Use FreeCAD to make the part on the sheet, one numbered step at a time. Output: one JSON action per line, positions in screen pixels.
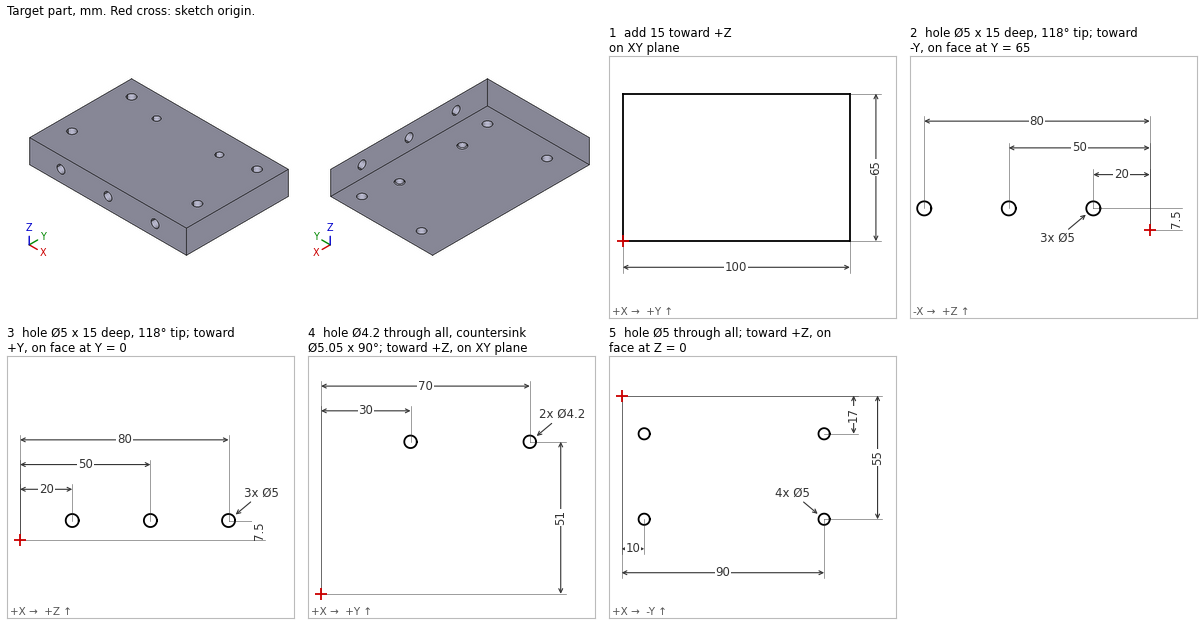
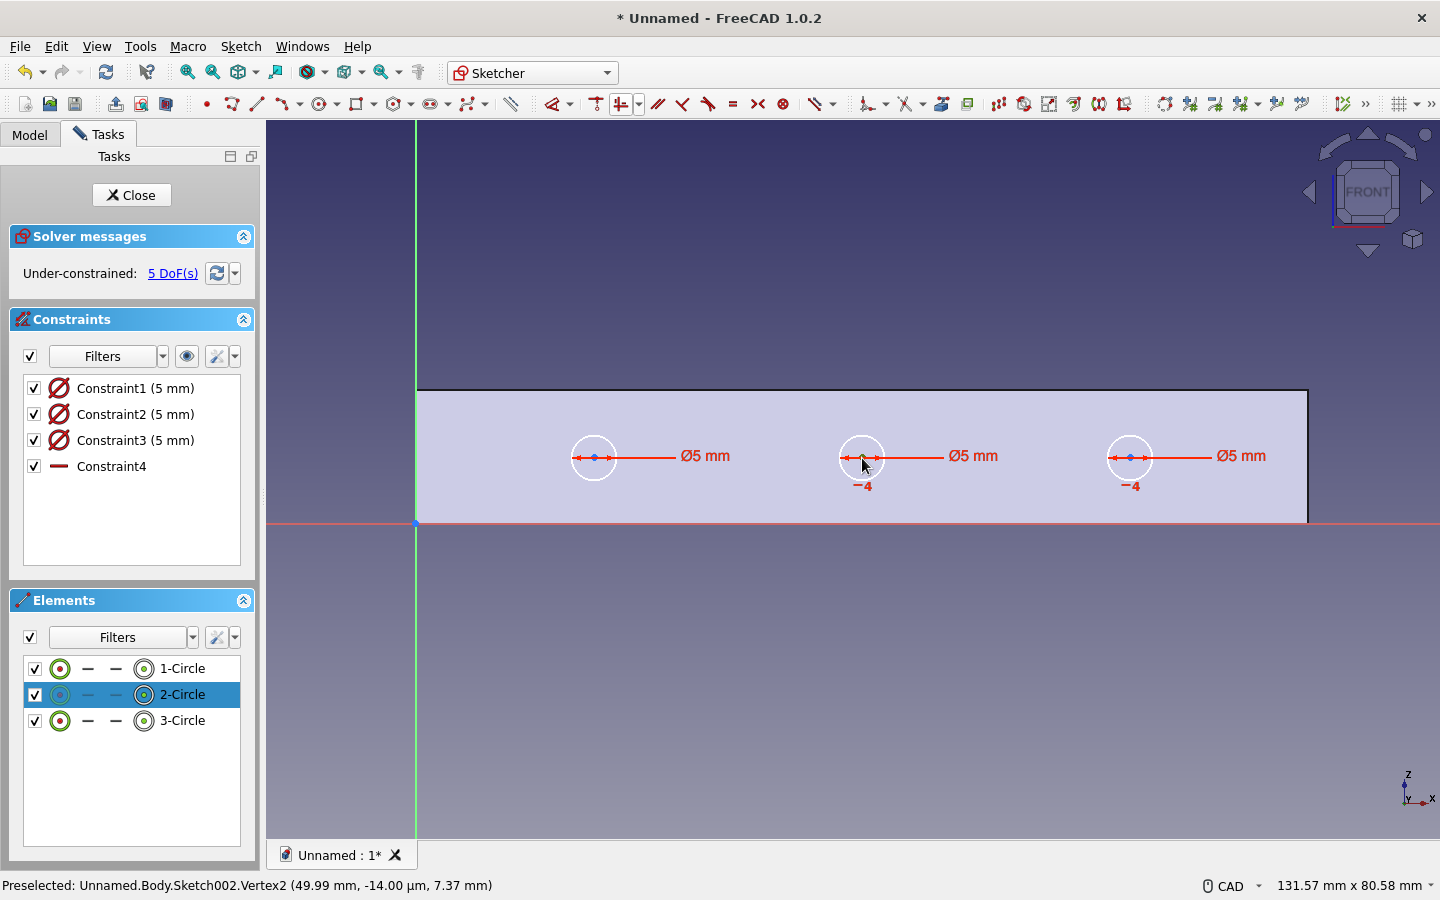
{"action": "left_click", "coordinate": [594, 458]}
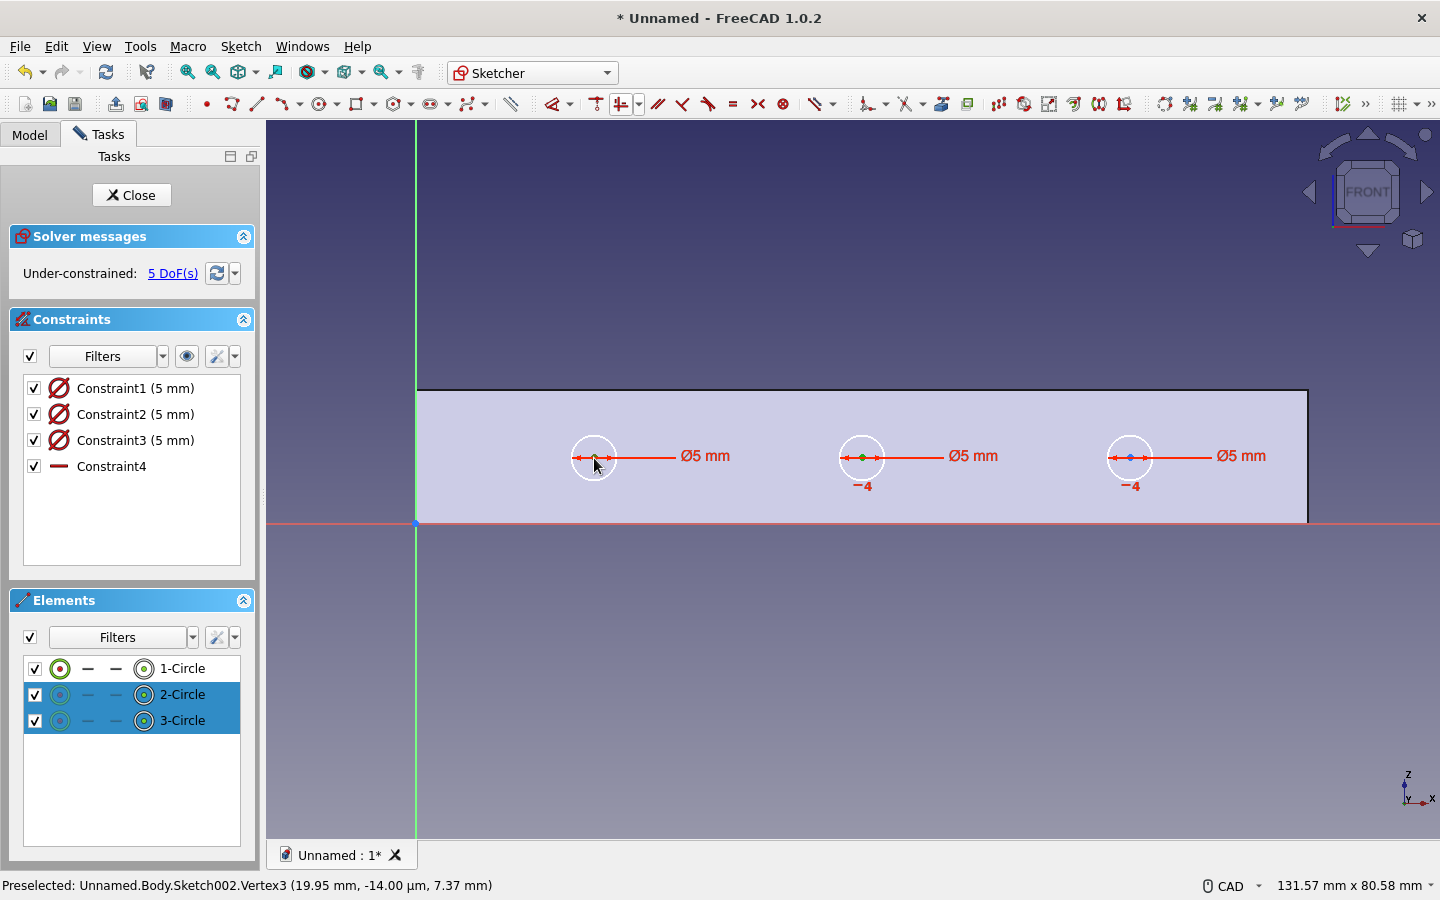
{"action": "key", "text": "h"}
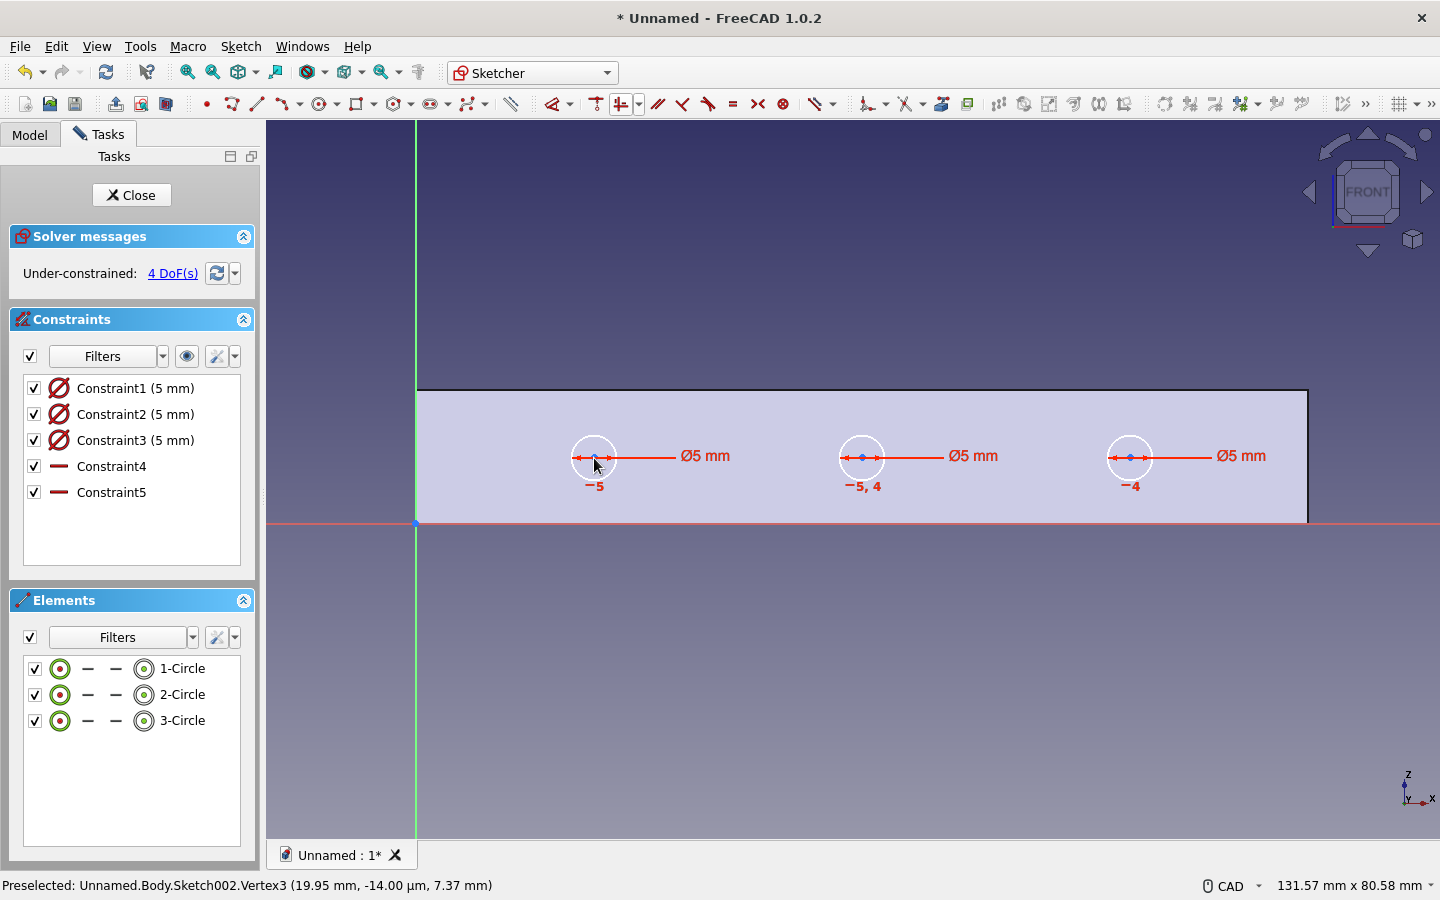
{"action": "left_click", "coordinate": [552, 104]}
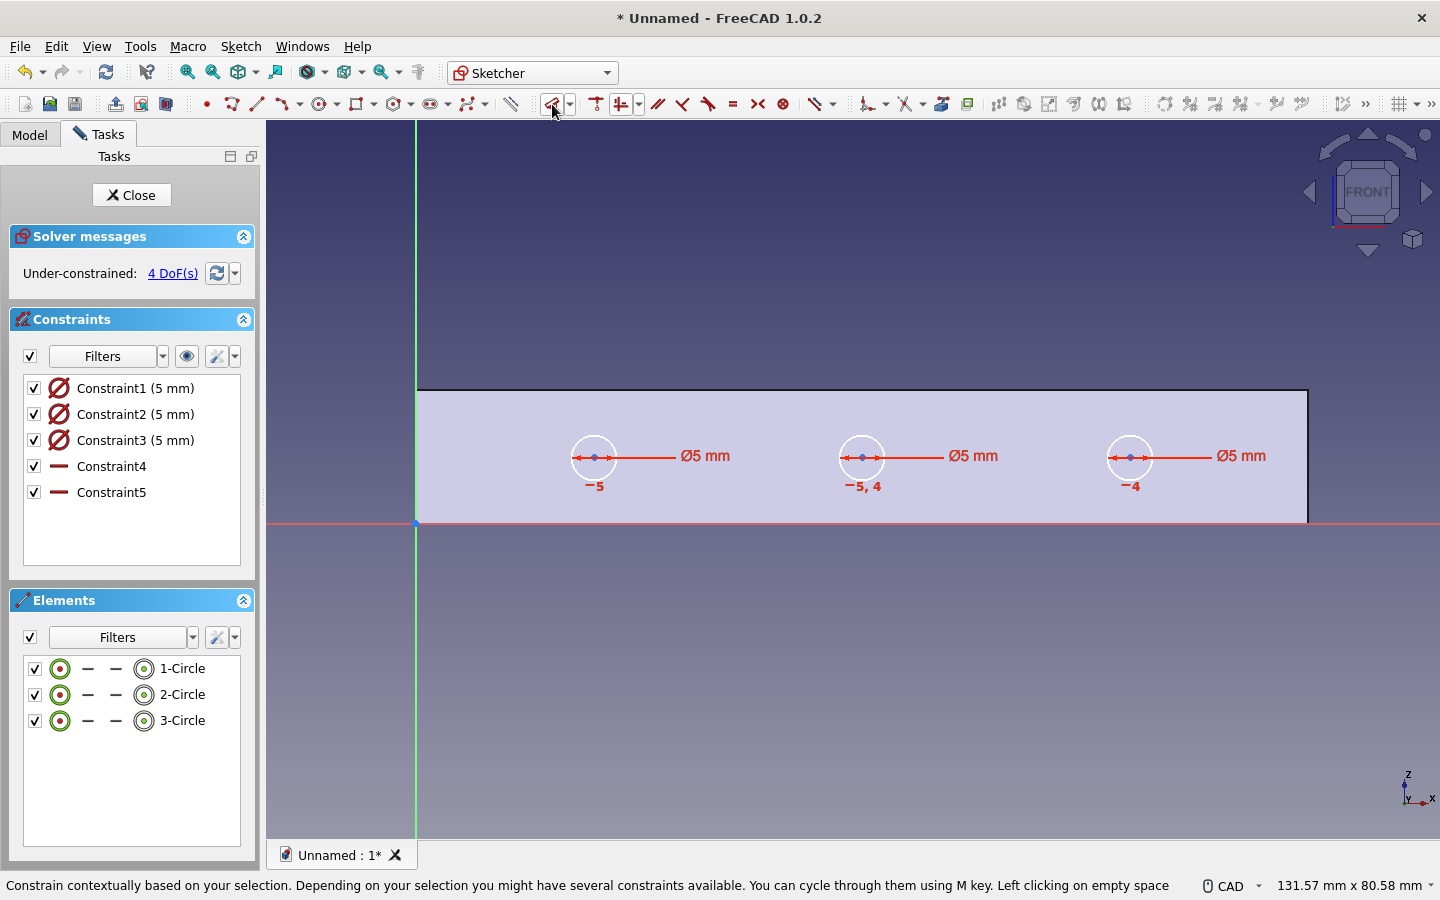
{"action": "left_click", "coordinate": [1130, 458]}
{"action": "left_click", "coordinate": [773, 558]}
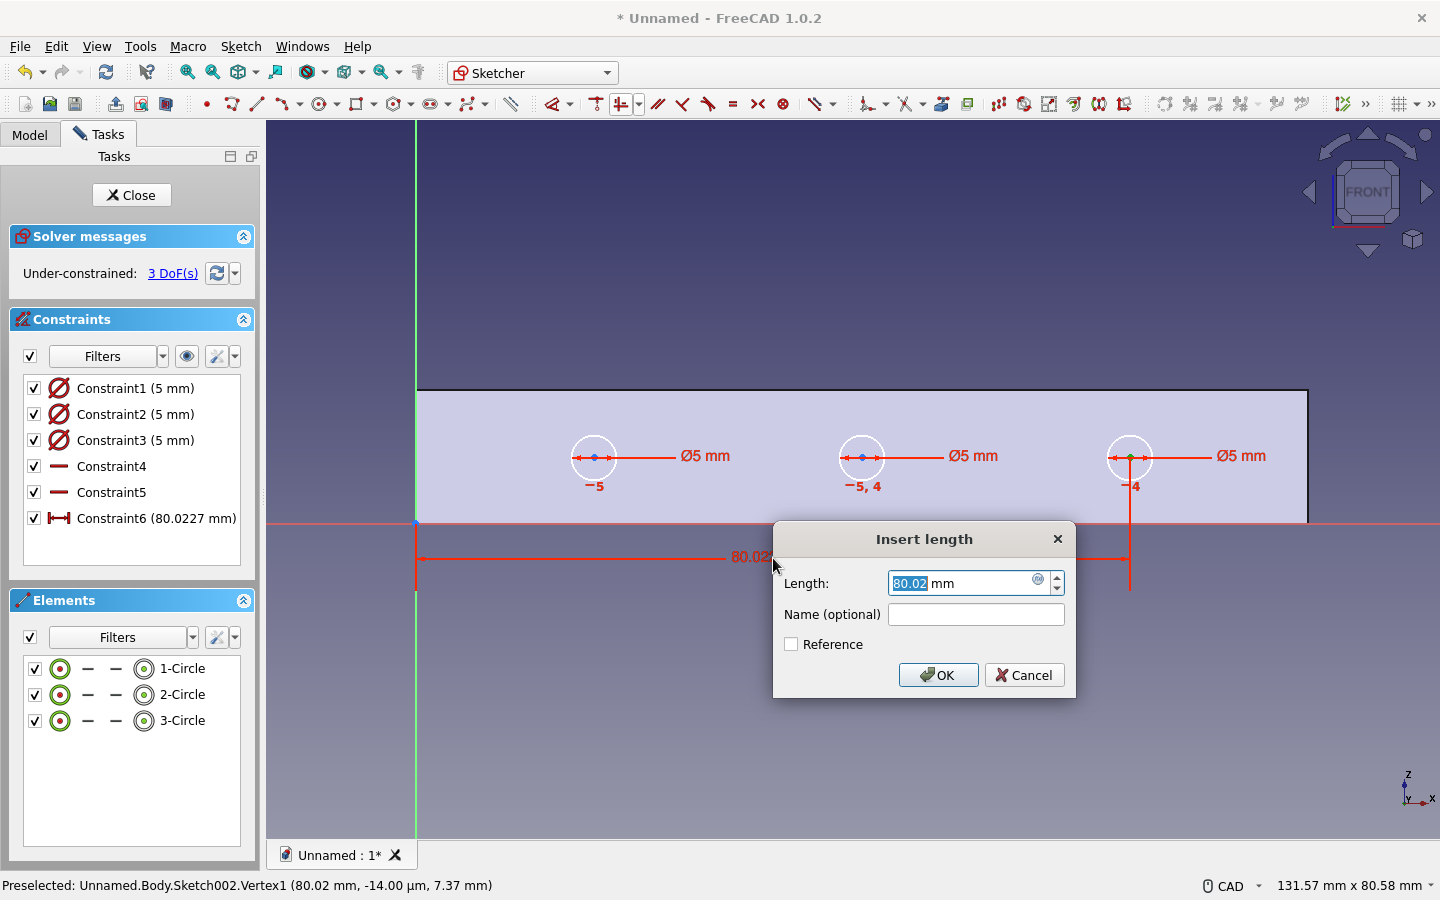
{"action": "type", "text": "80"}
{"action": "key", "text": "Return"}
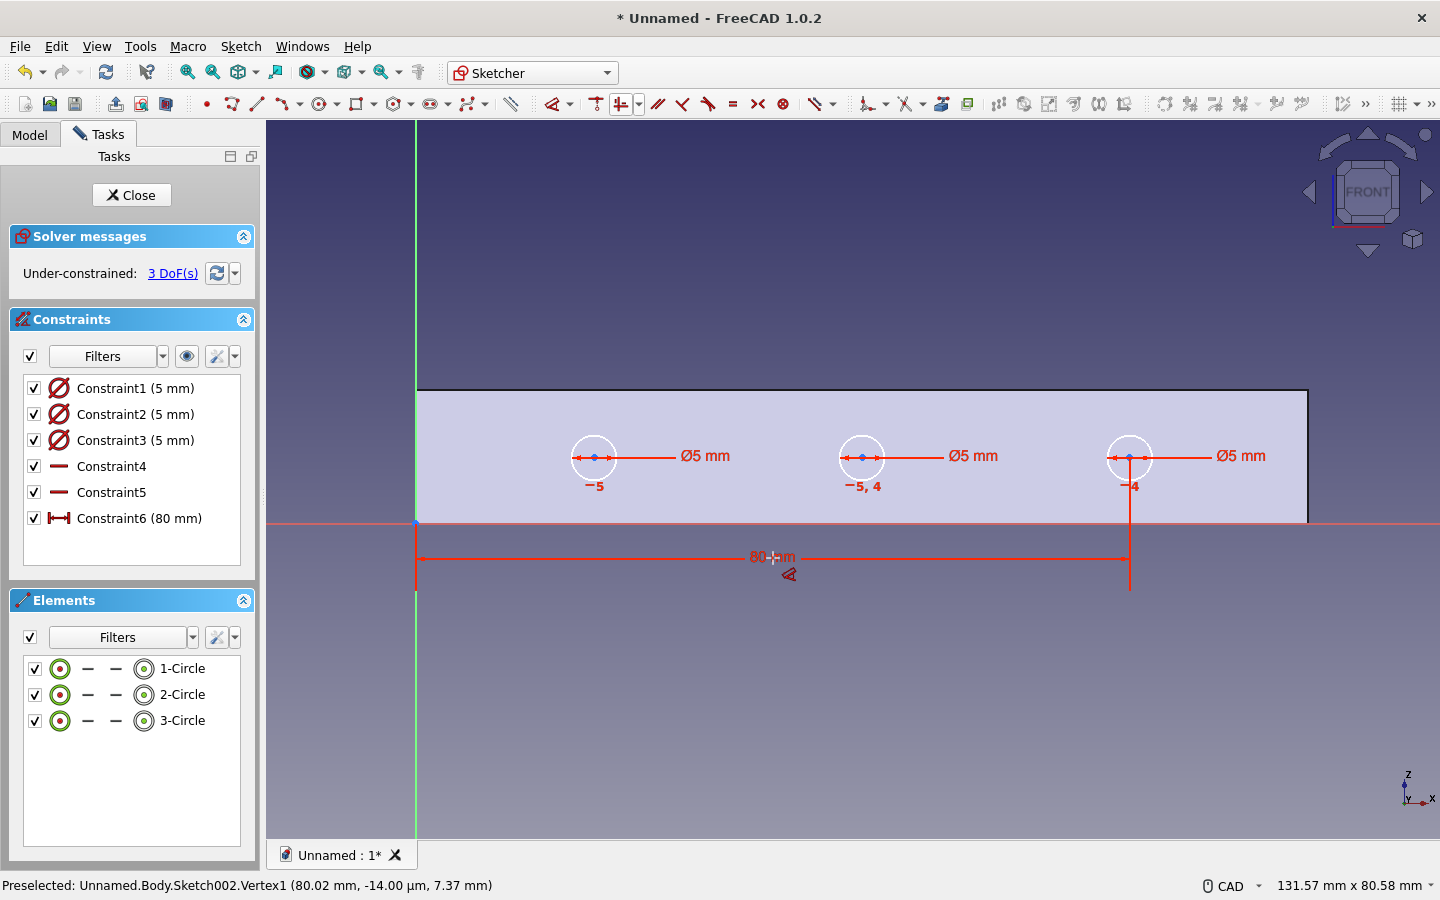
{"action": "left_click", "coordinate": [862, 458]}
{"action": "left_click", "coordinate": [639, 558]}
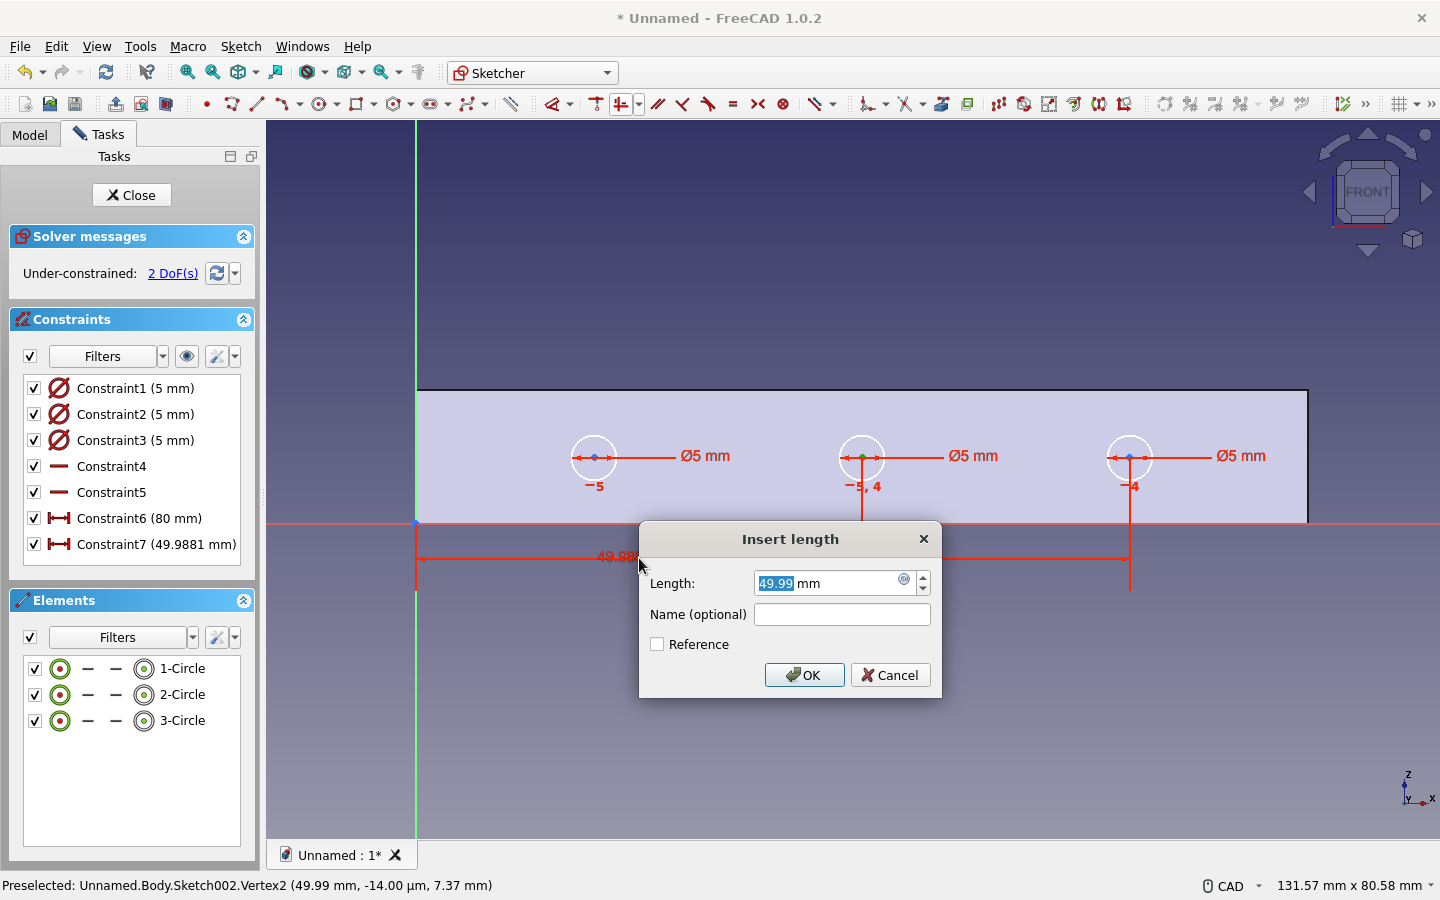
{"action": "type", "text": "50"}
{"action": "key", "text": "Return"}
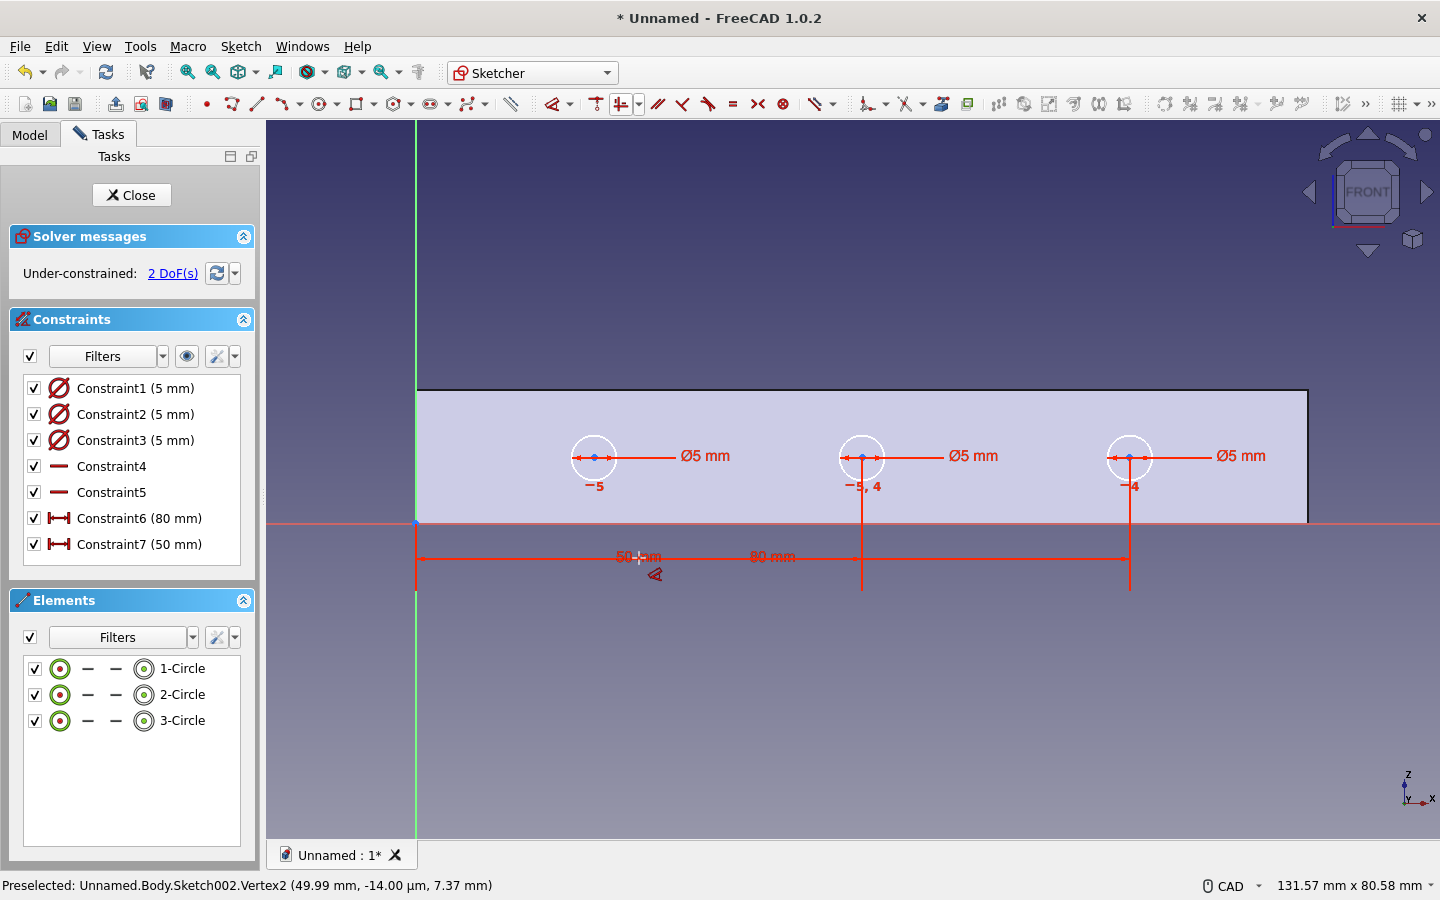
{"action": "left_click", "coordinate": [594, 458]}
{"action": "left_click", "coordinate": [505, 558]}